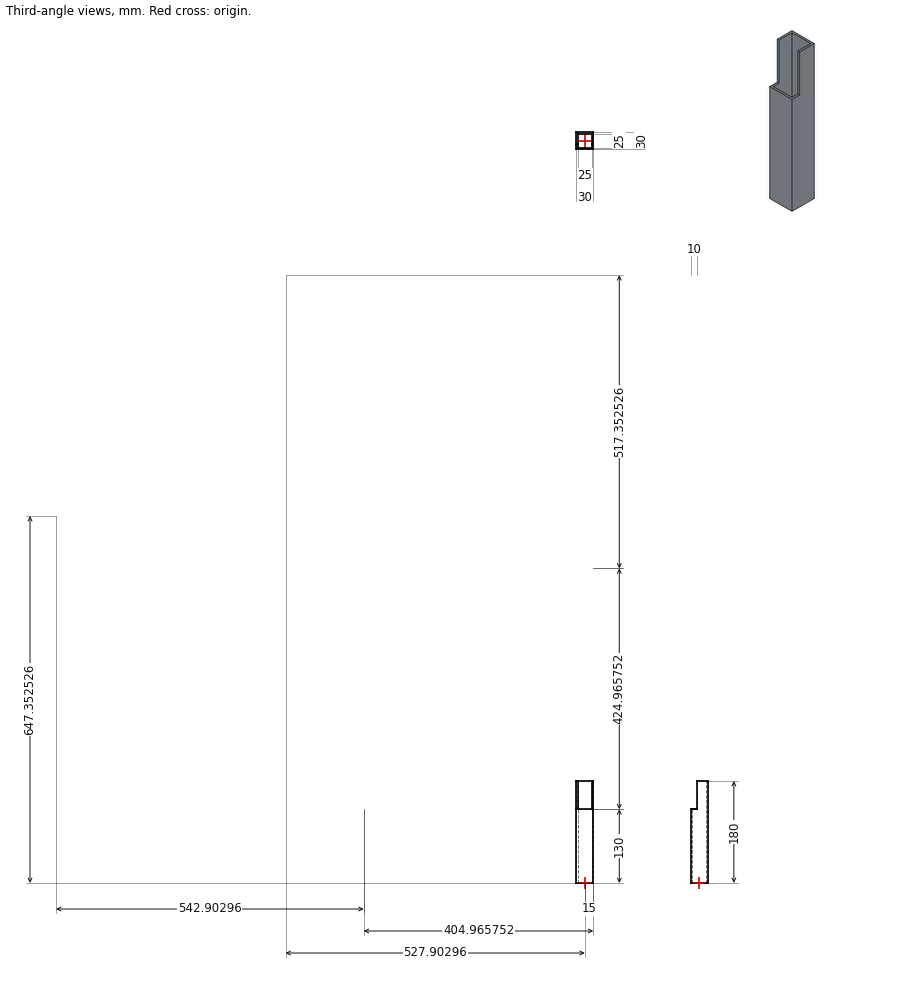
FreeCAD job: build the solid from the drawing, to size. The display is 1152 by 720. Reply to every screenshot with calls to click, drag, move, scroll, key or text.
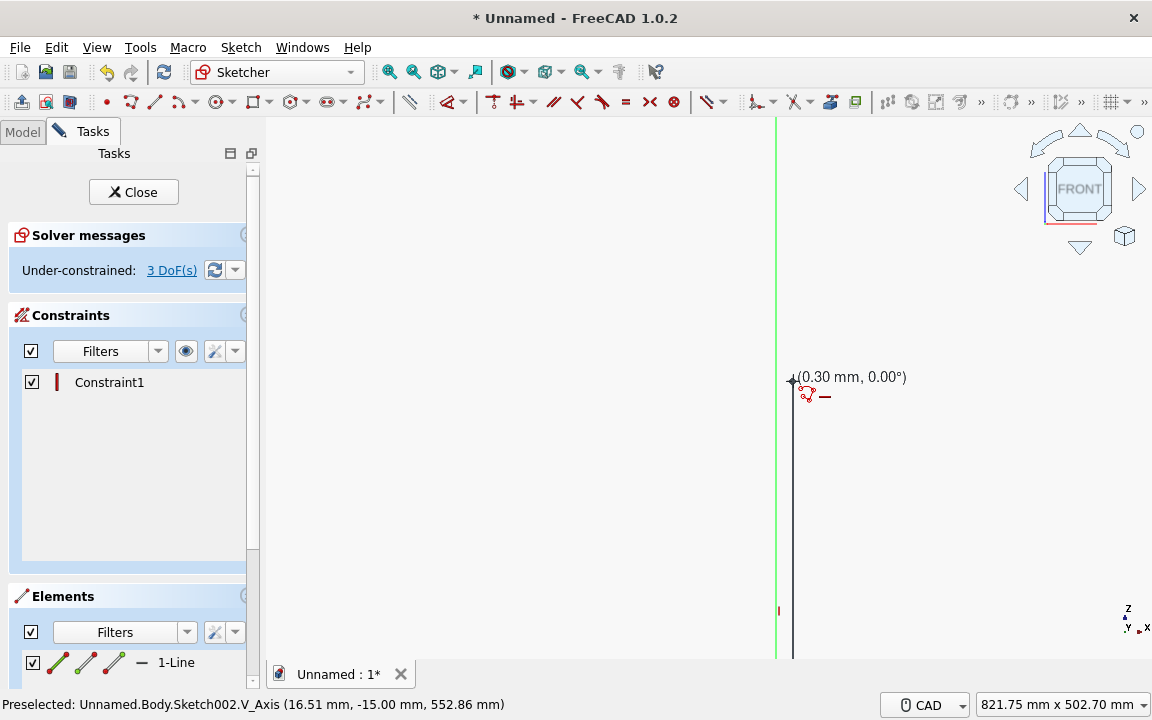
scroll(795, 382, down, 6)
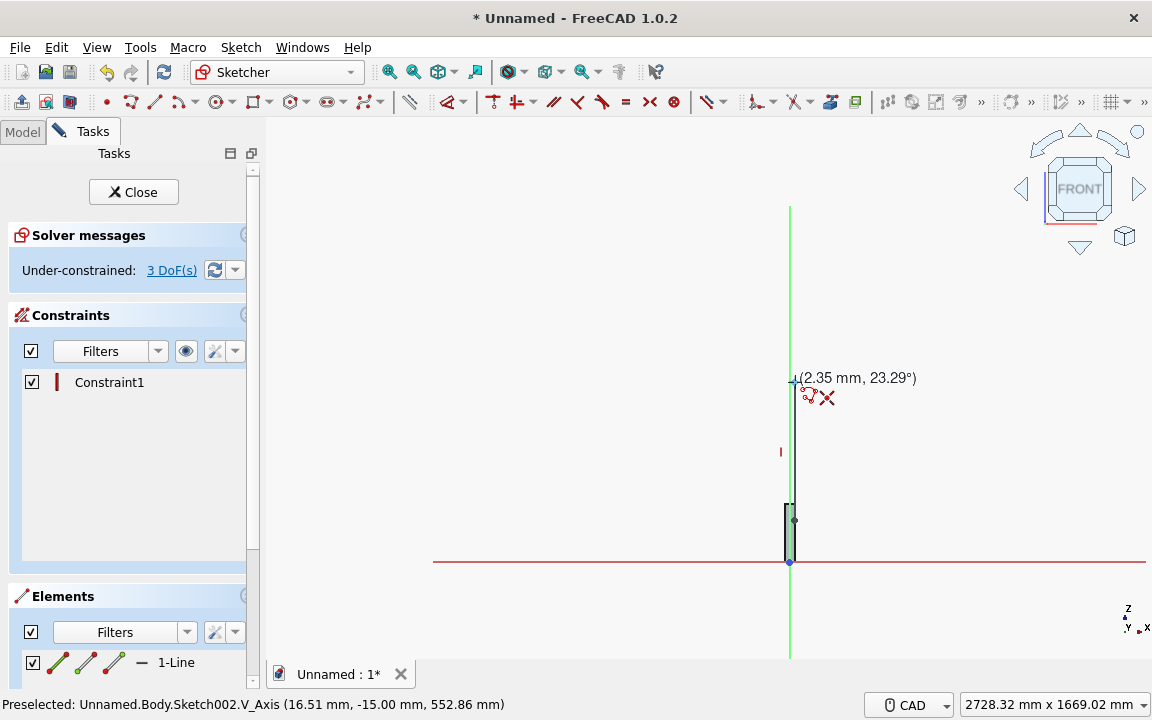
click(618, 214)
click(487, 352)
click(663, 520)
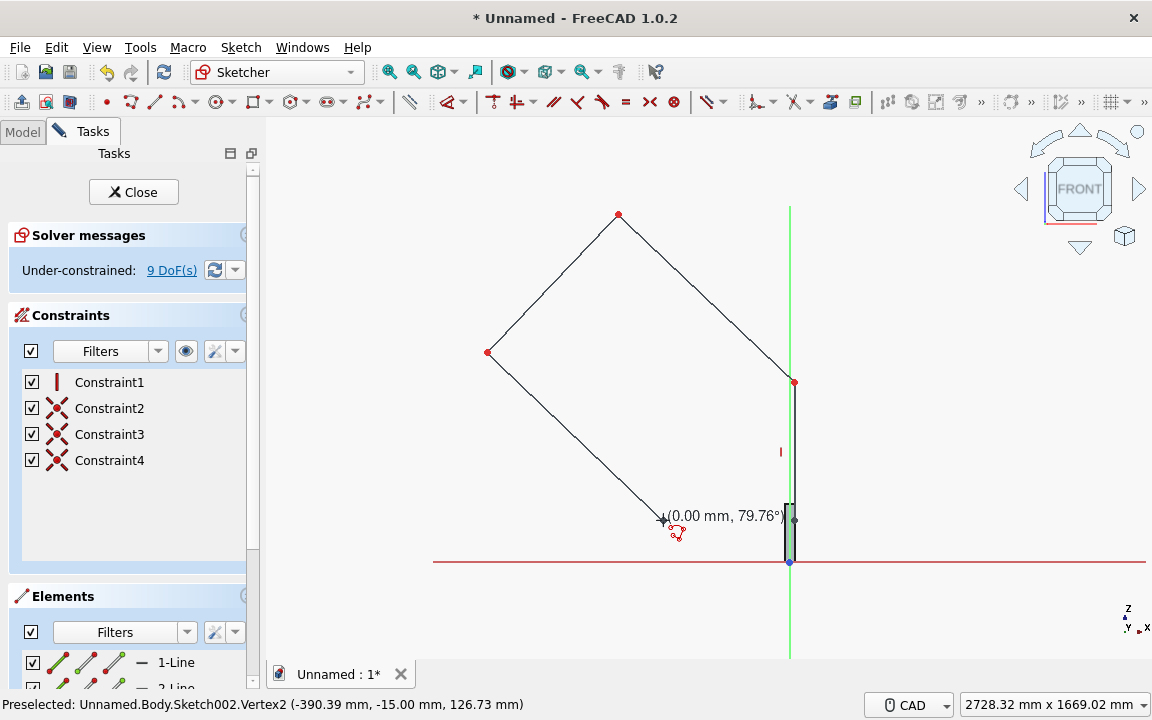
scroll(795, 520, up, 6)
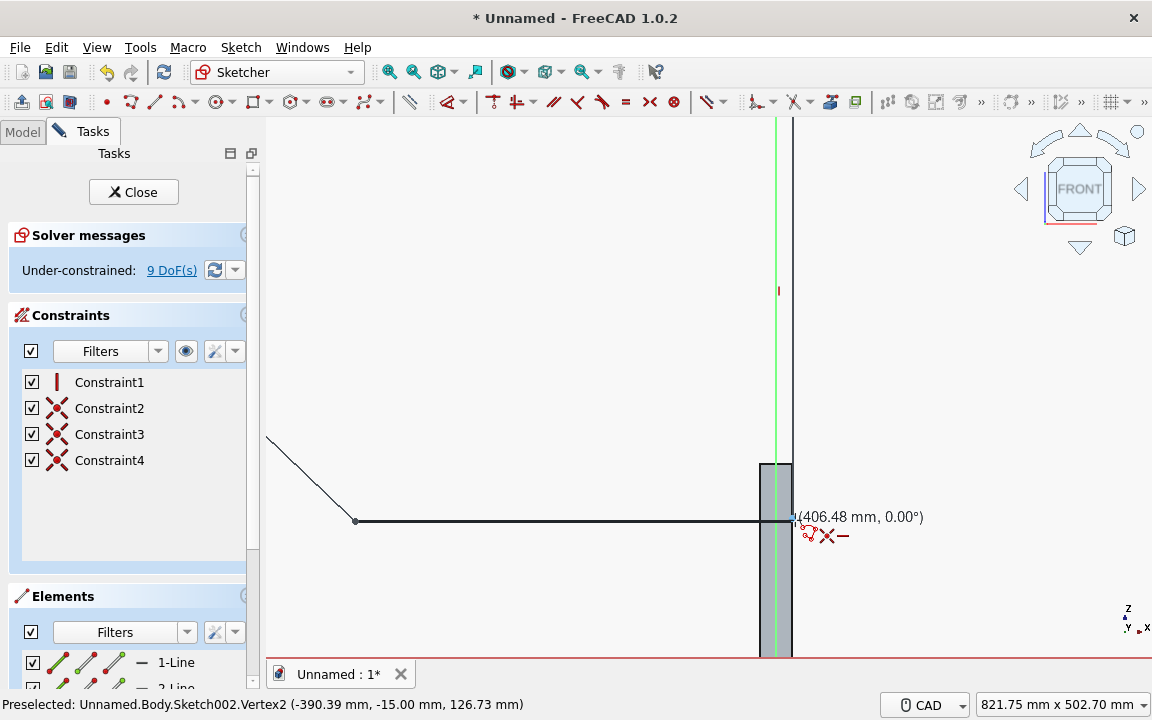
click(793, 519)
key(Escape)
key(Escape)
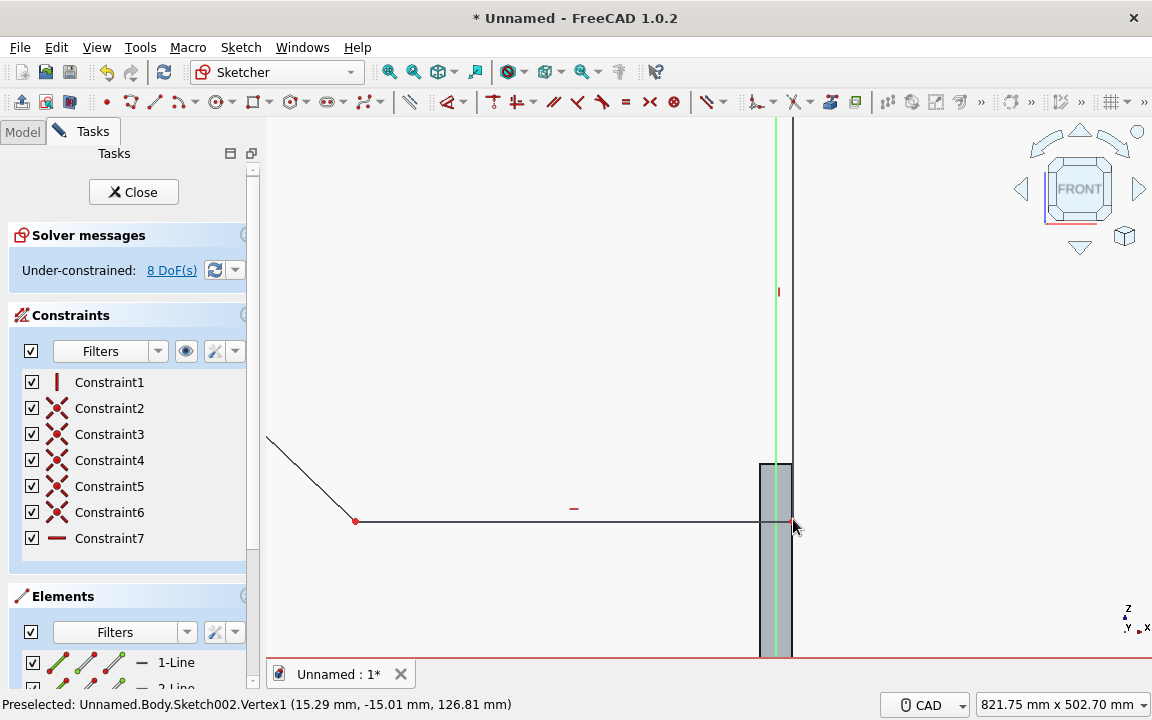
scroll(793, 522, up, 5)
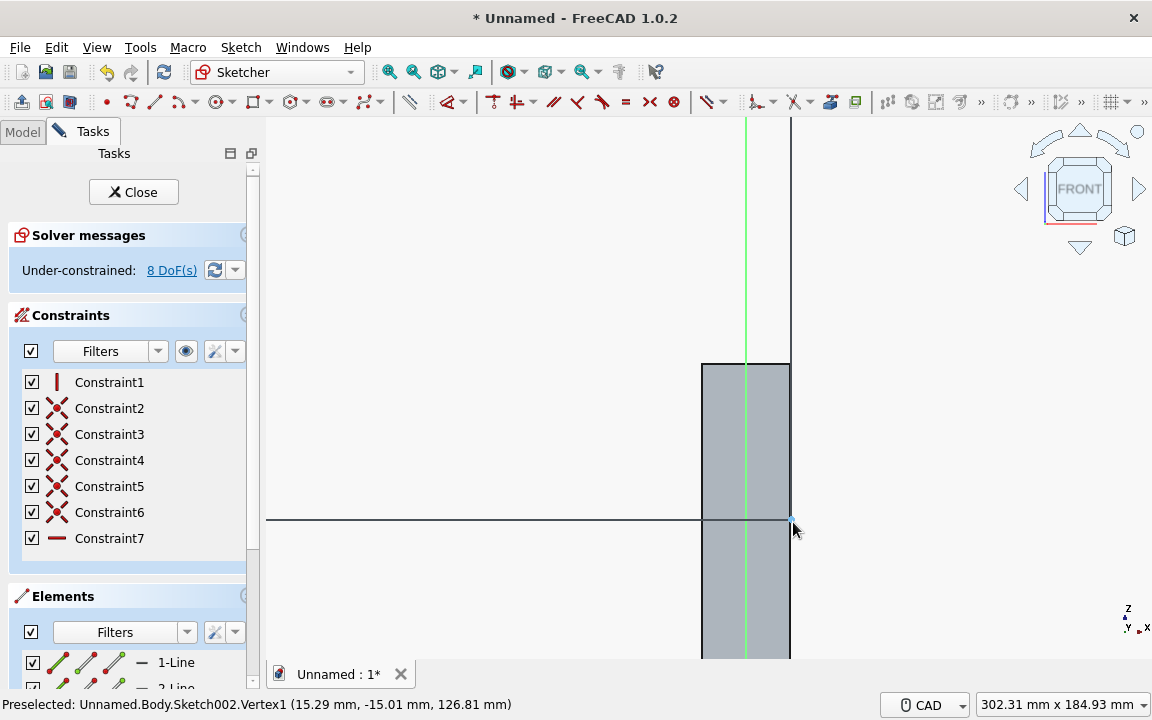
click(791, 520)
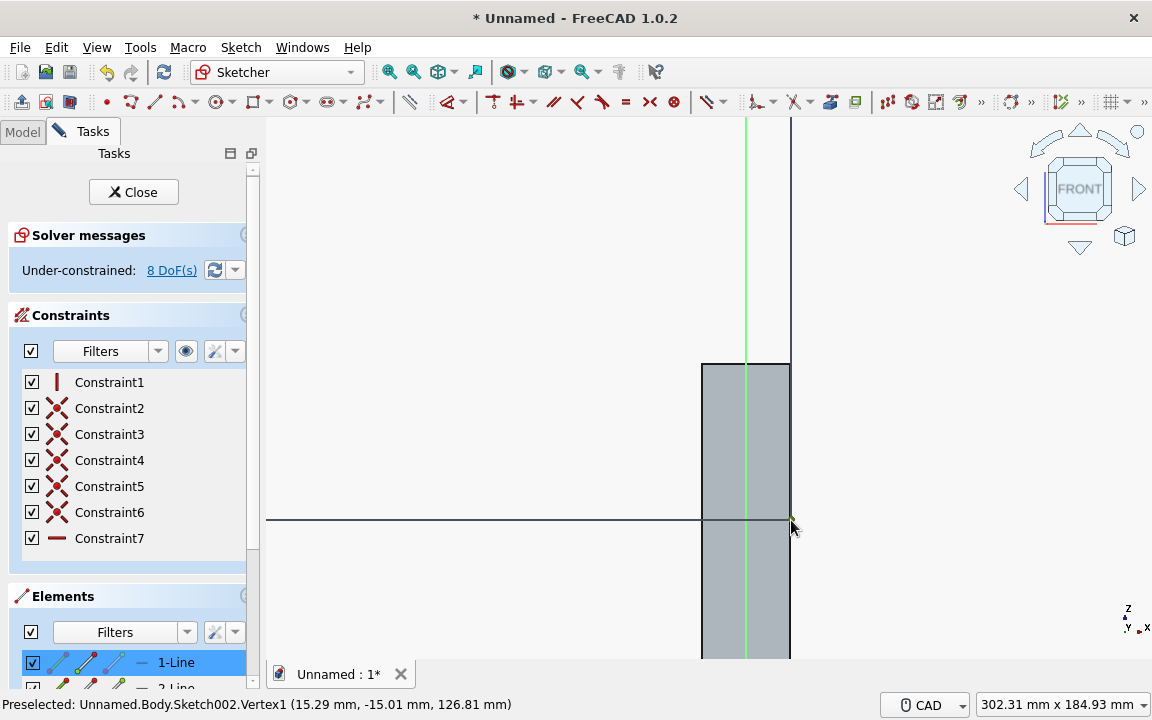
key(l)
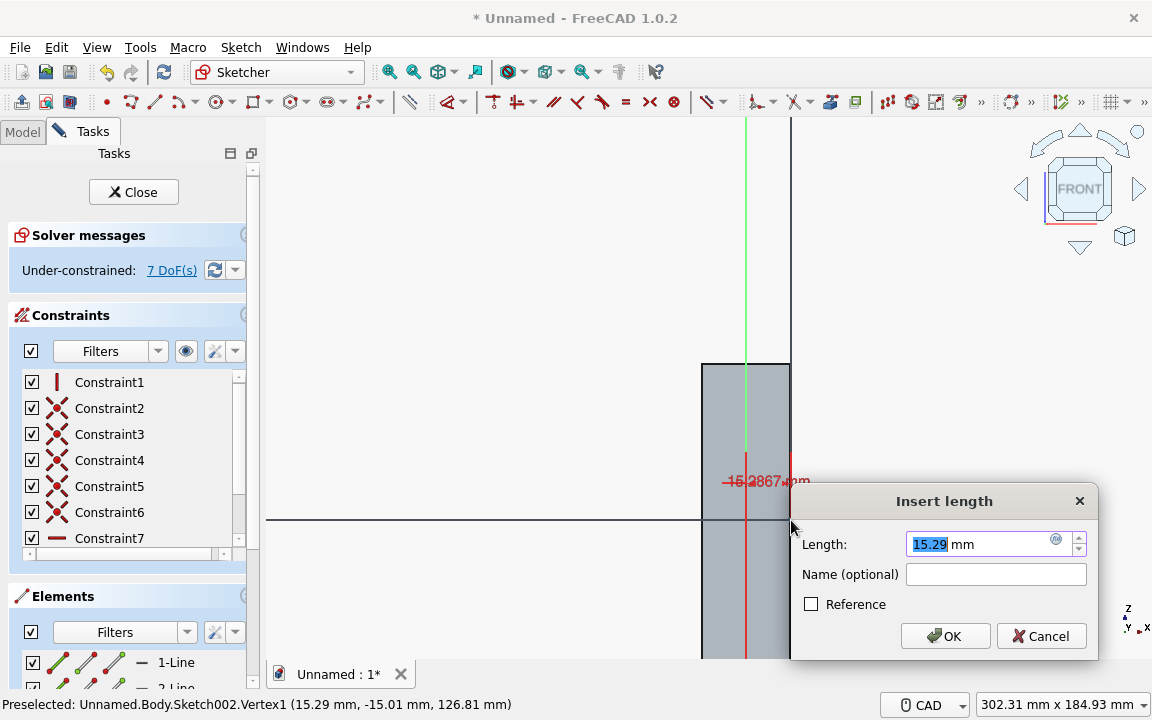
text(15)
key(Return)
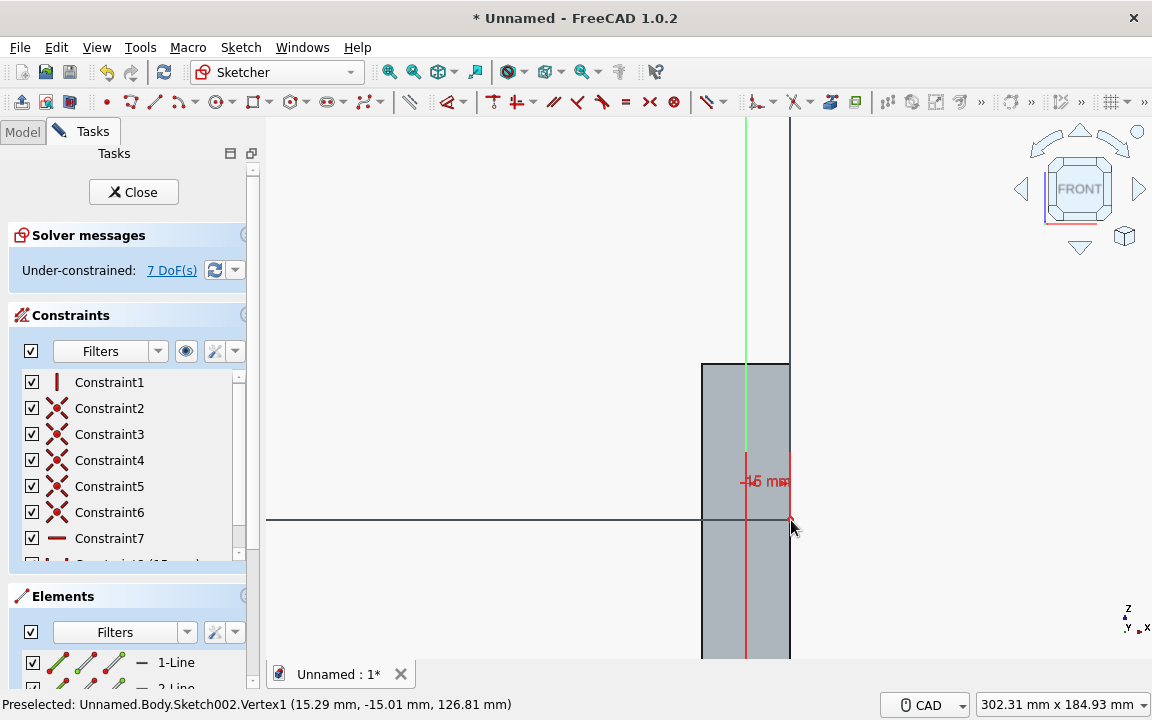
scroll(795, 521, down, 11)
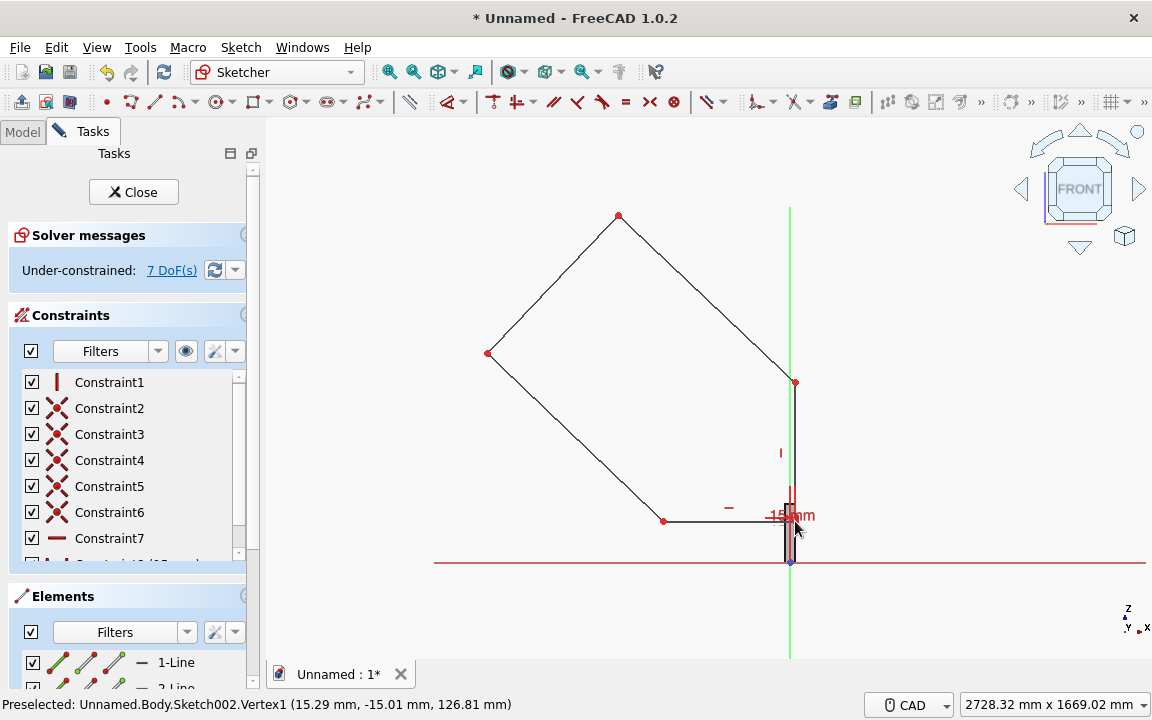
click(795, 522)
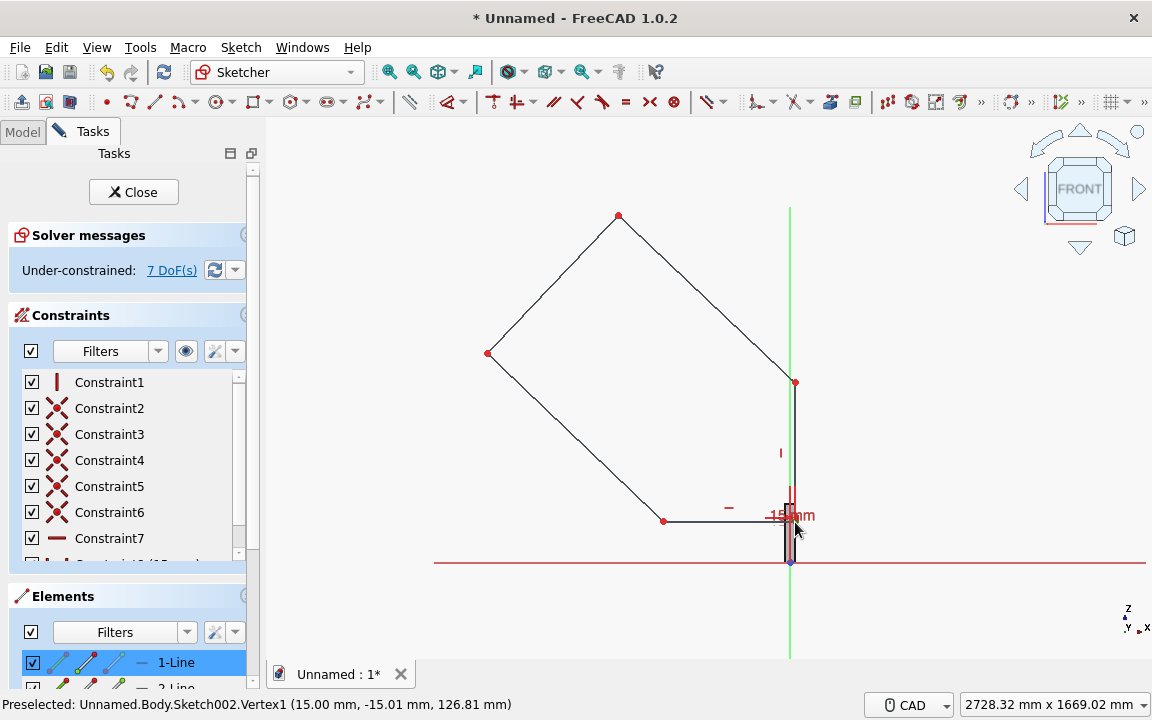
key(i)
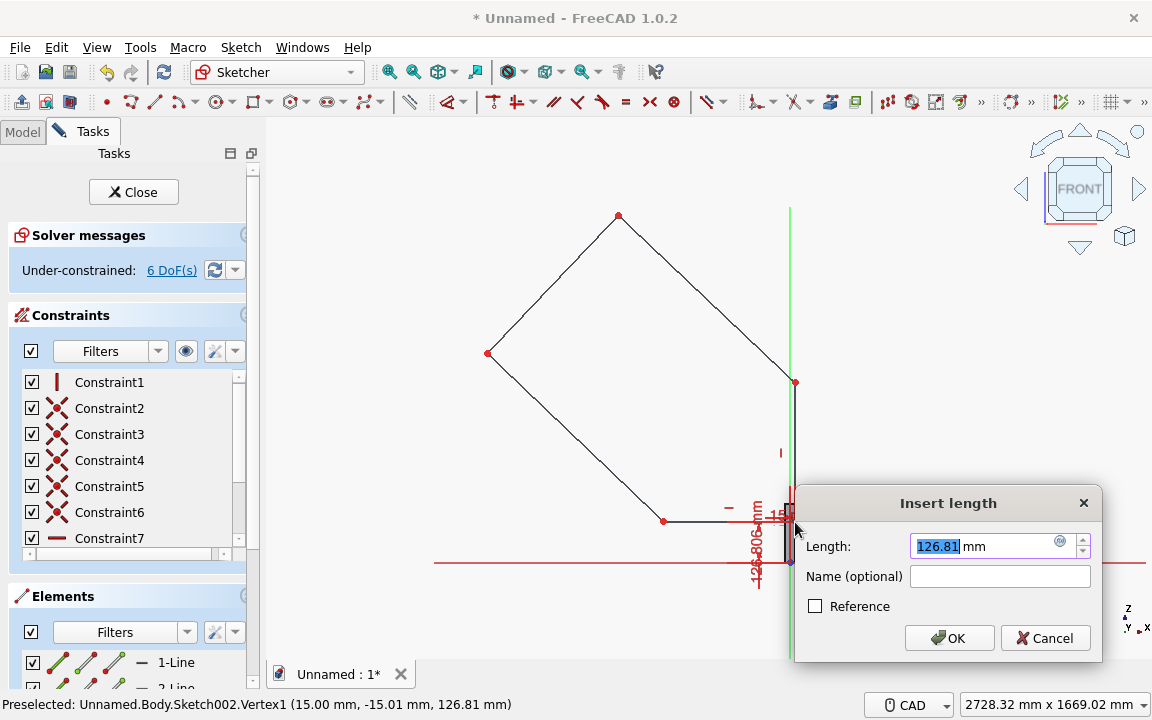
text(130)
key(Return)